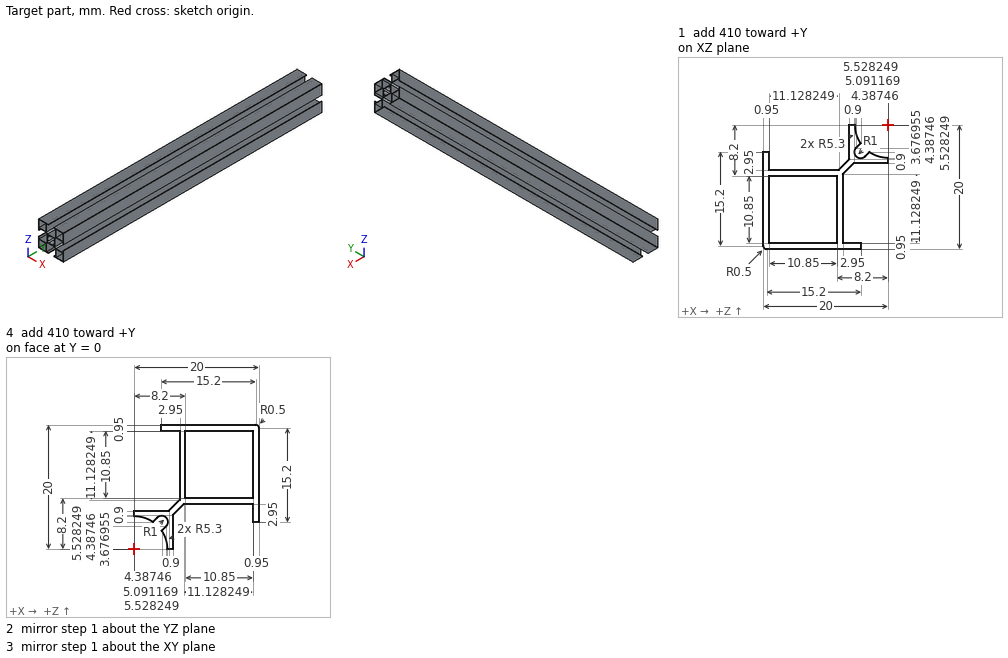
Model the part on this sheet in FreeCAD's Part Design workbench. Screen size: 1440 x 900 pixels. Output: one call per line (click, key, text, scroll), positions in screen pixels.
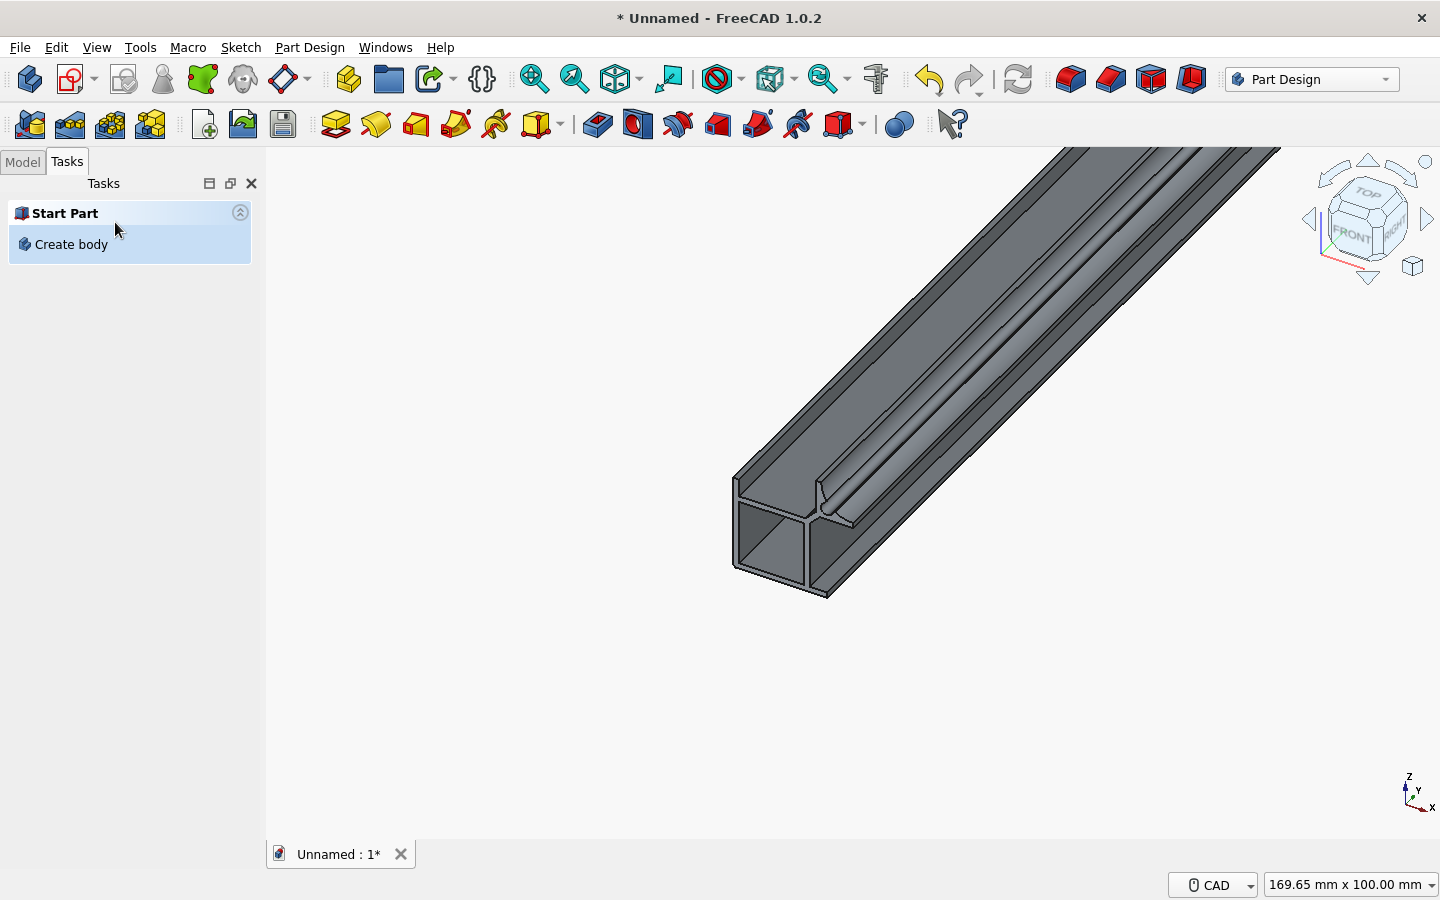
click(536, 80)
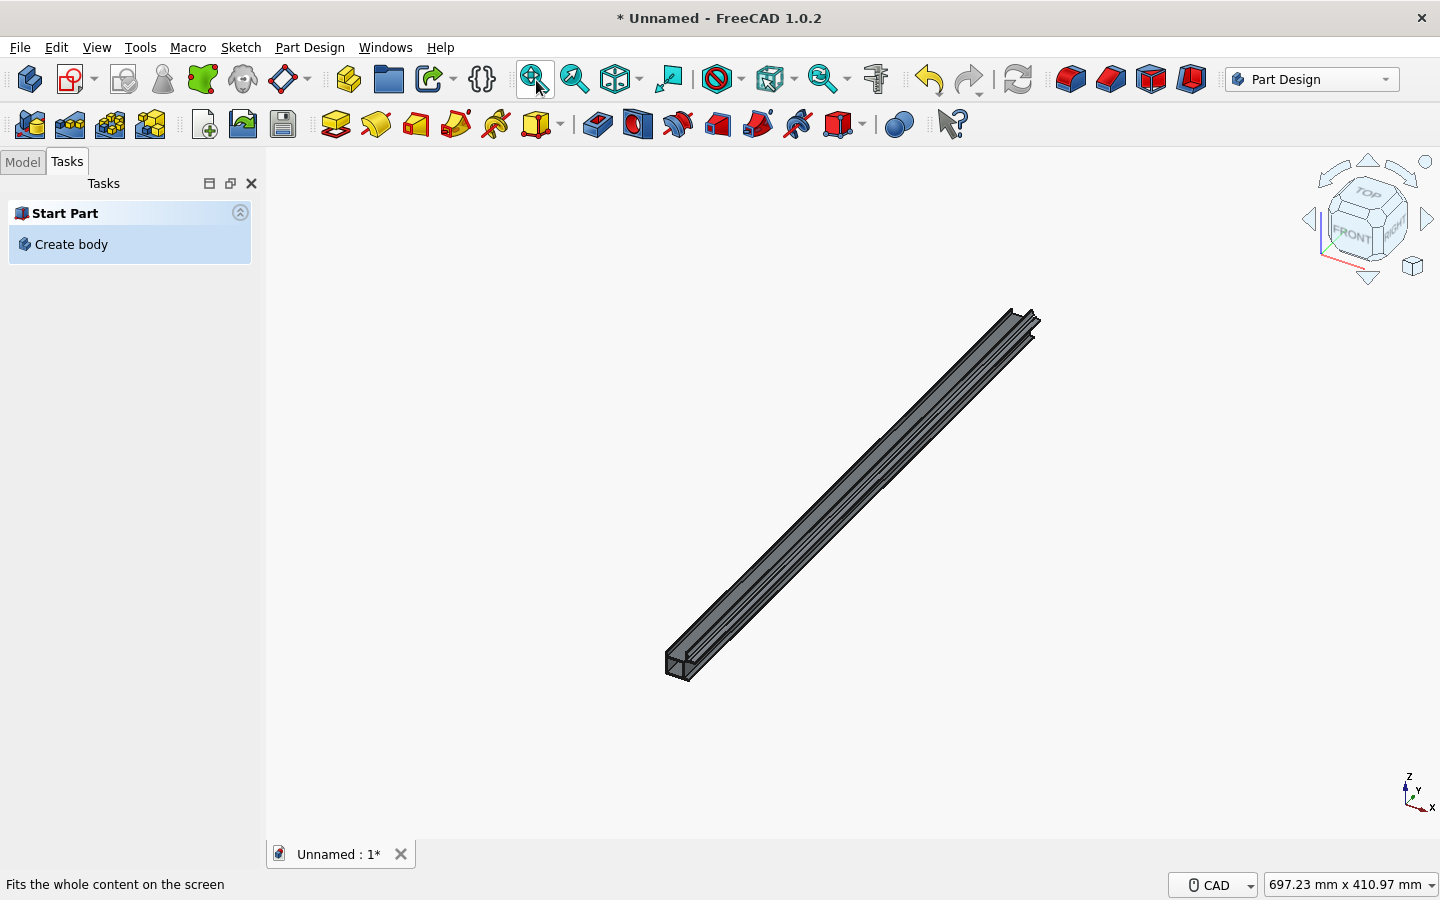
click(23, 161)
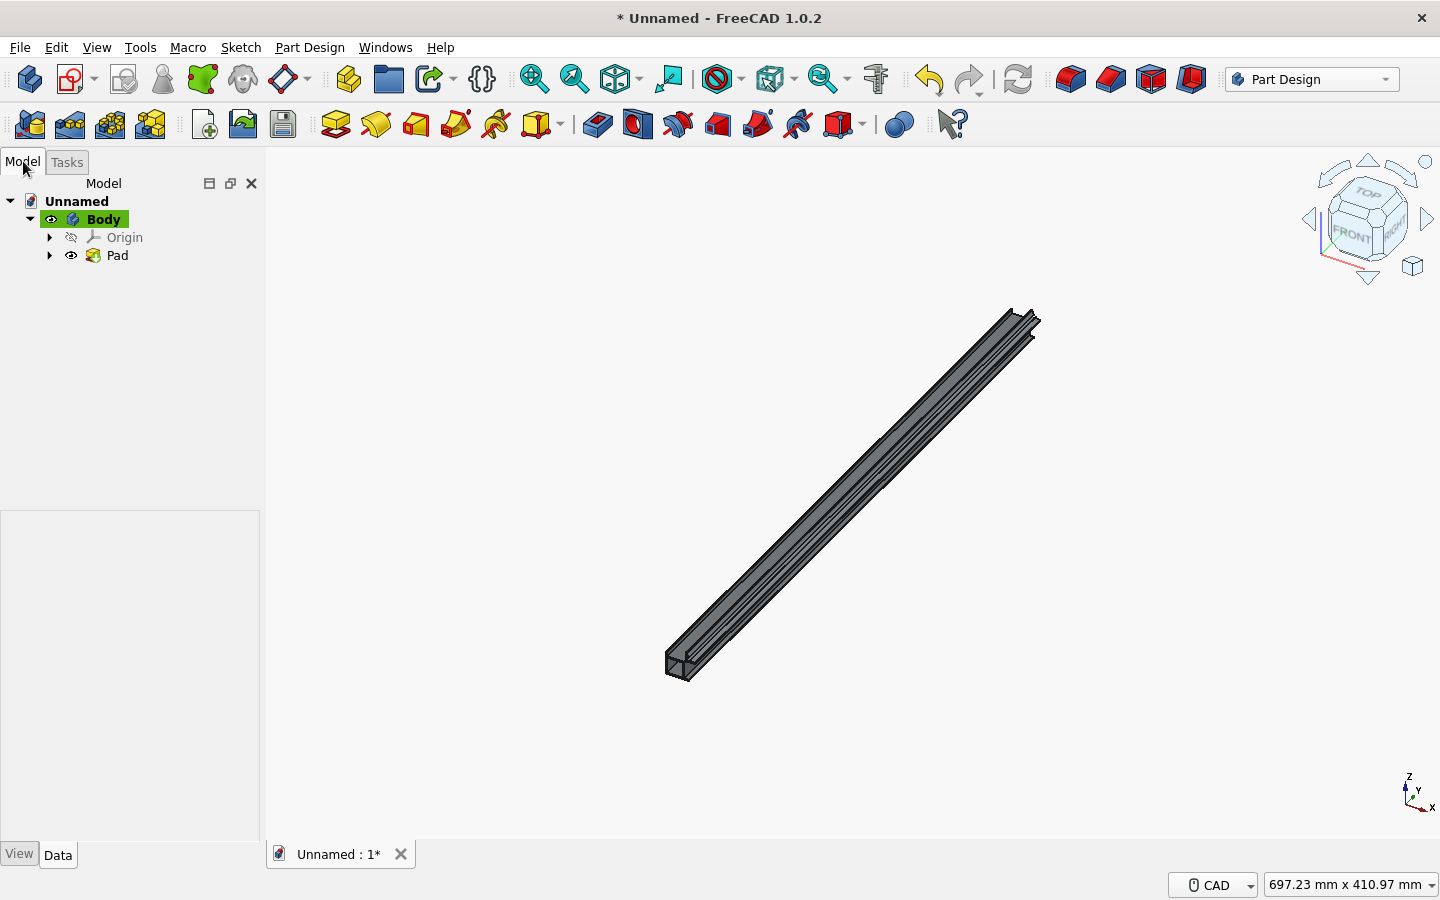
click(116, 255)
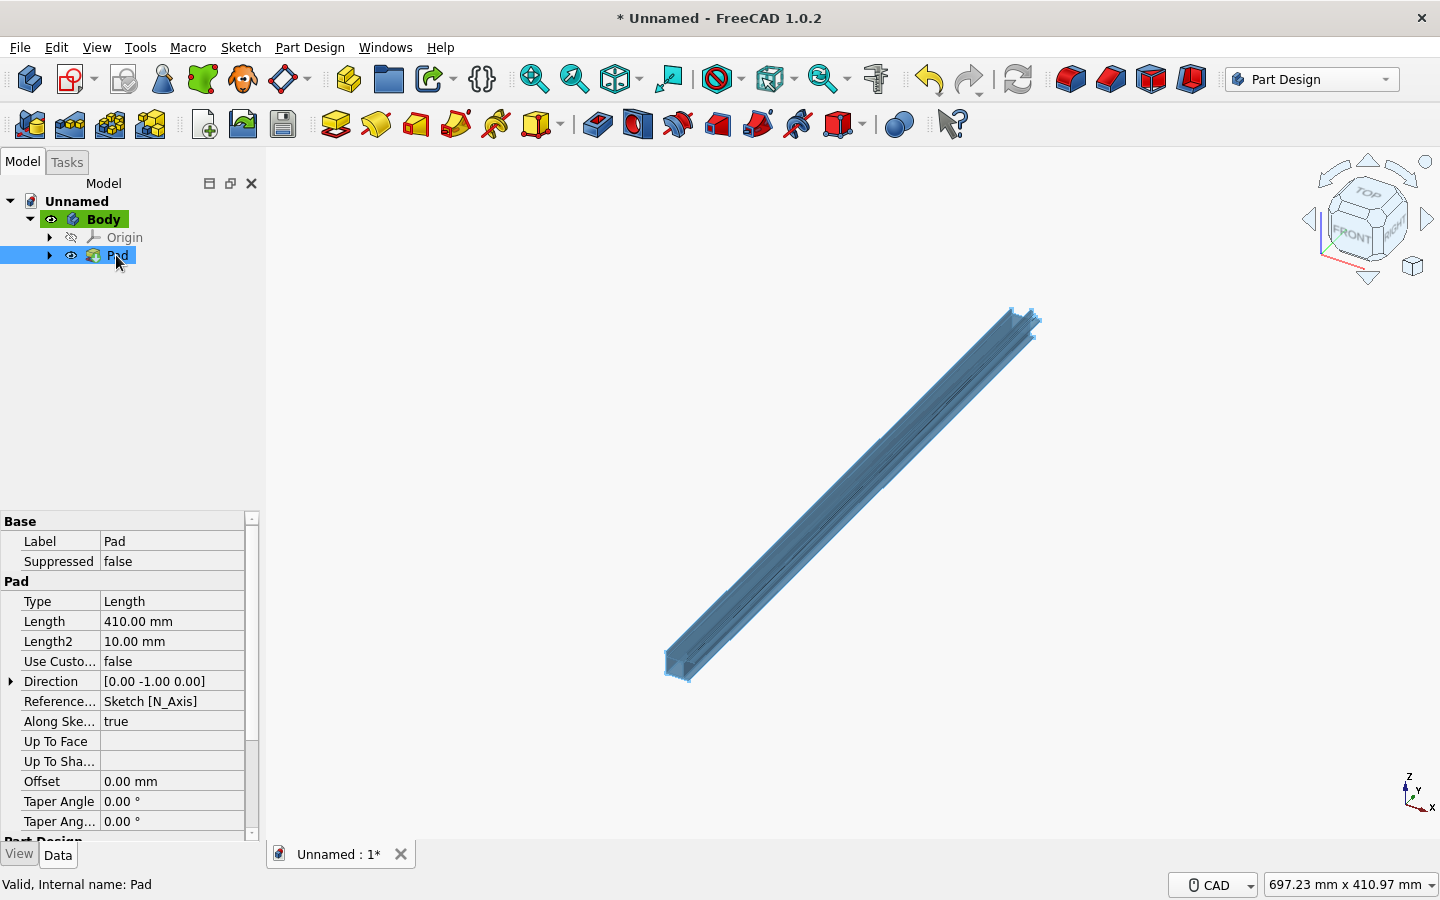
click(30, 124)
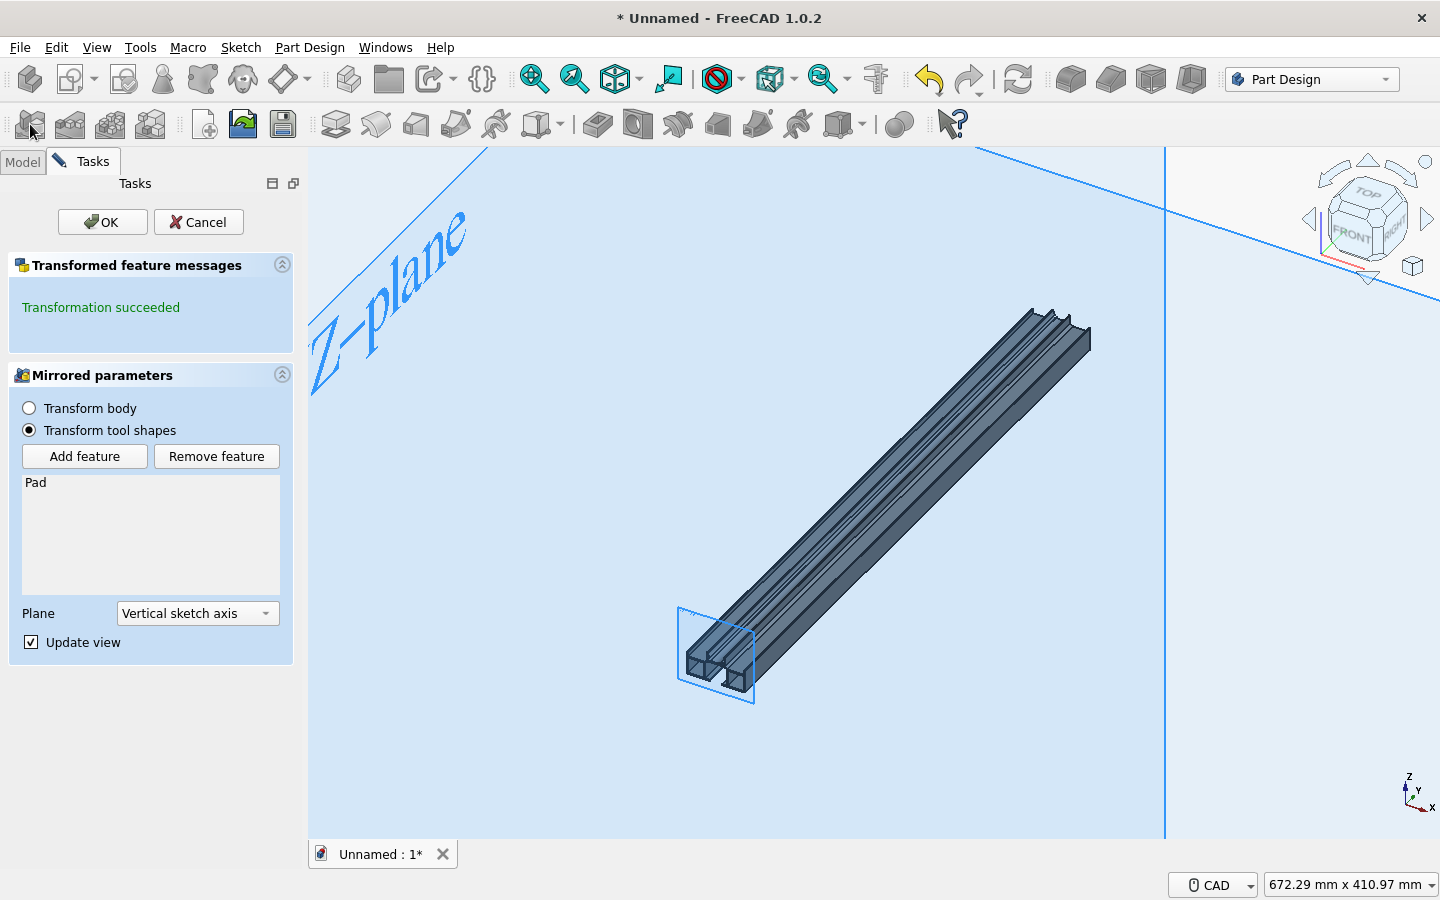
click(198, 614)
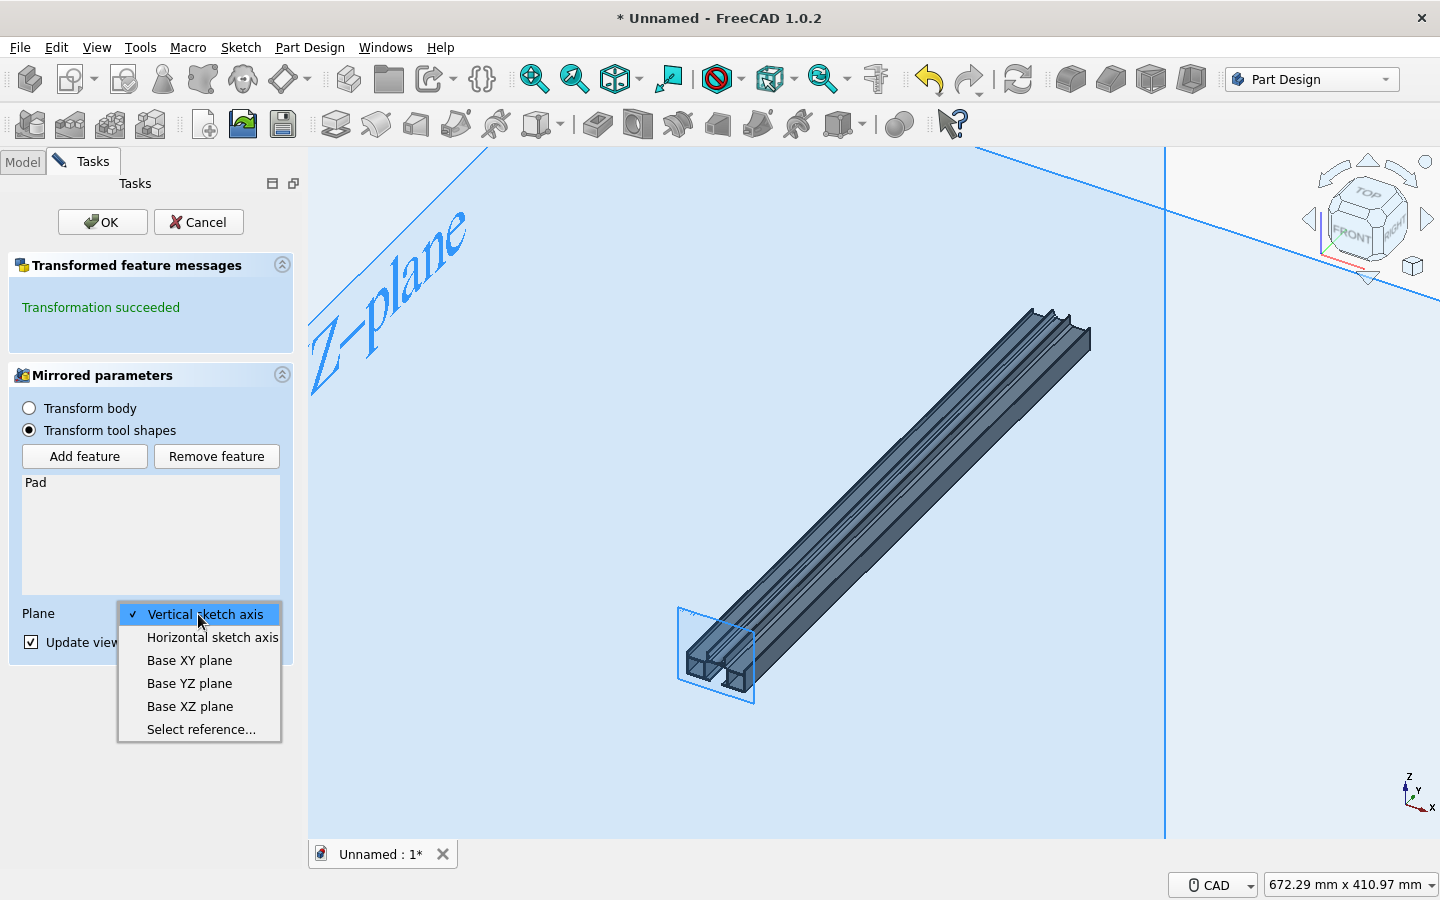
click(198, 684)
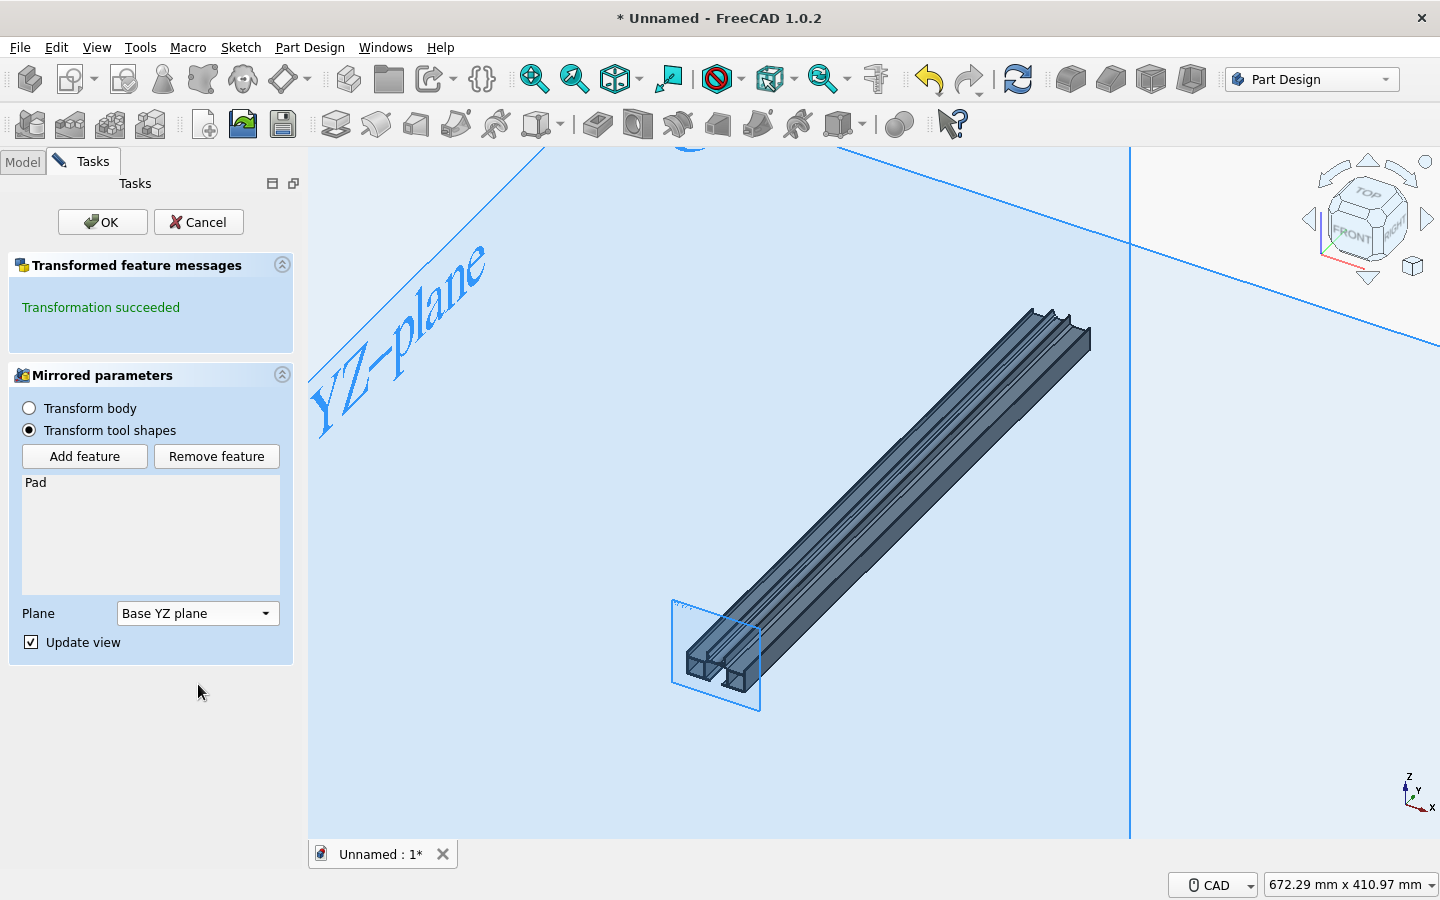
click(103, 222)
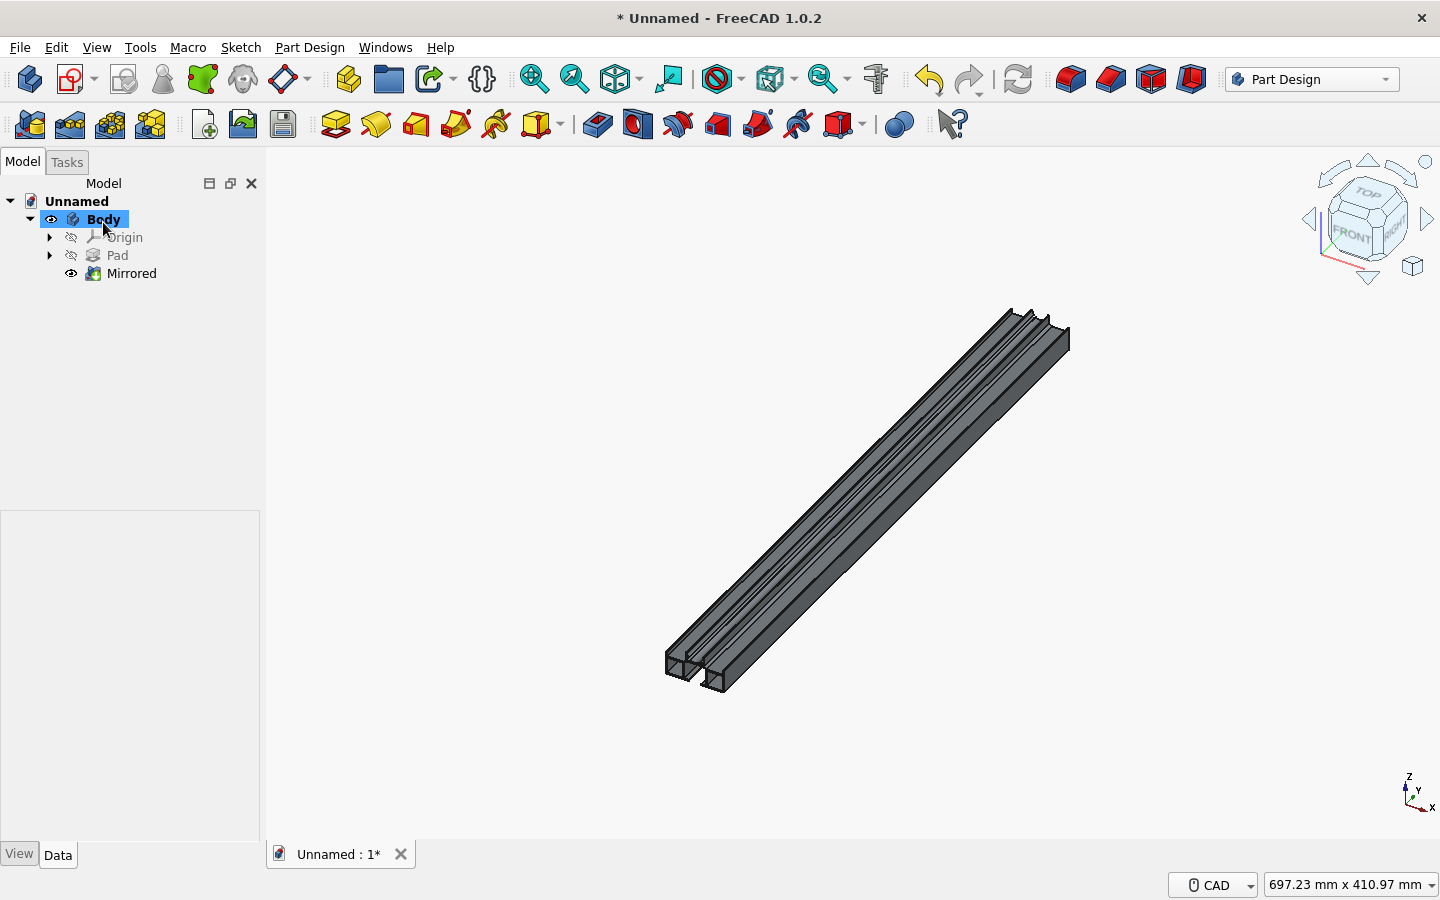
click(116, 255)